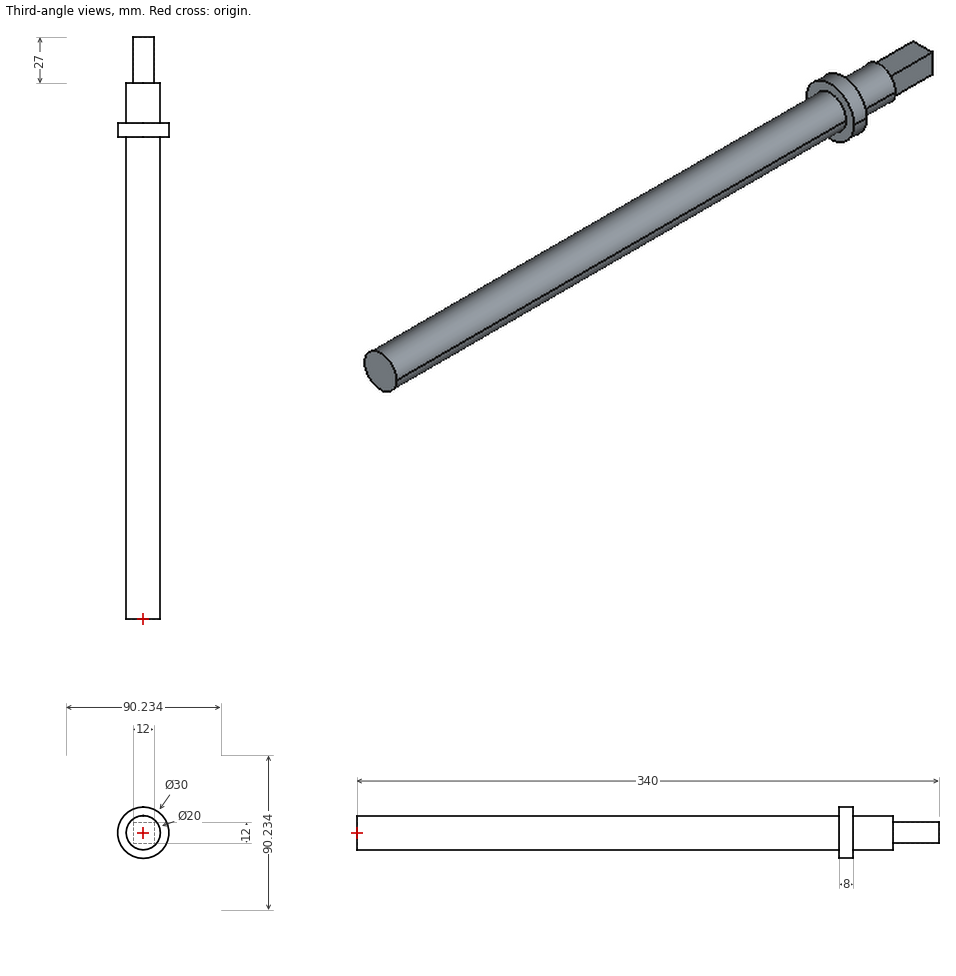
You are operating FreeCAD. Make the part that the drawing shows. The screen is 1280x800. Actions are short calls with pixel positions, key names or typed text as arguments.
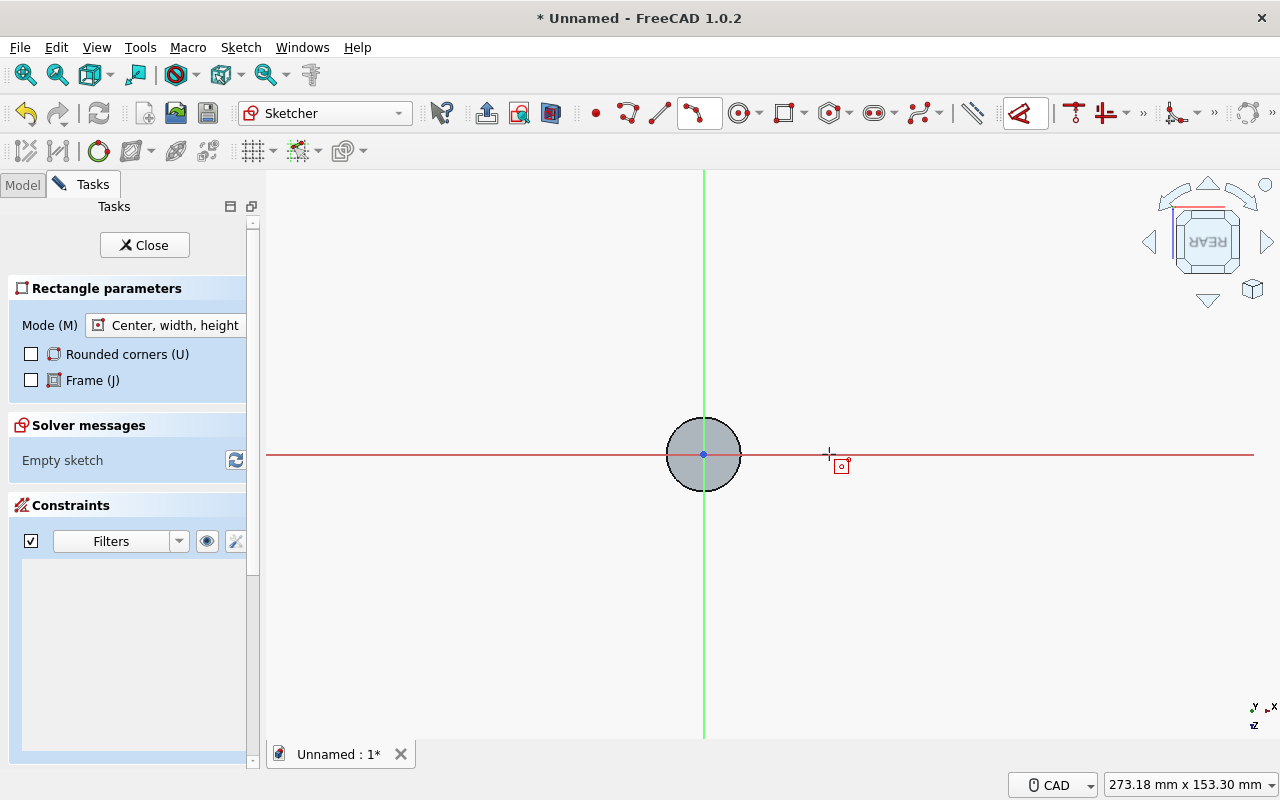
click(704, 454)
move(871, 287)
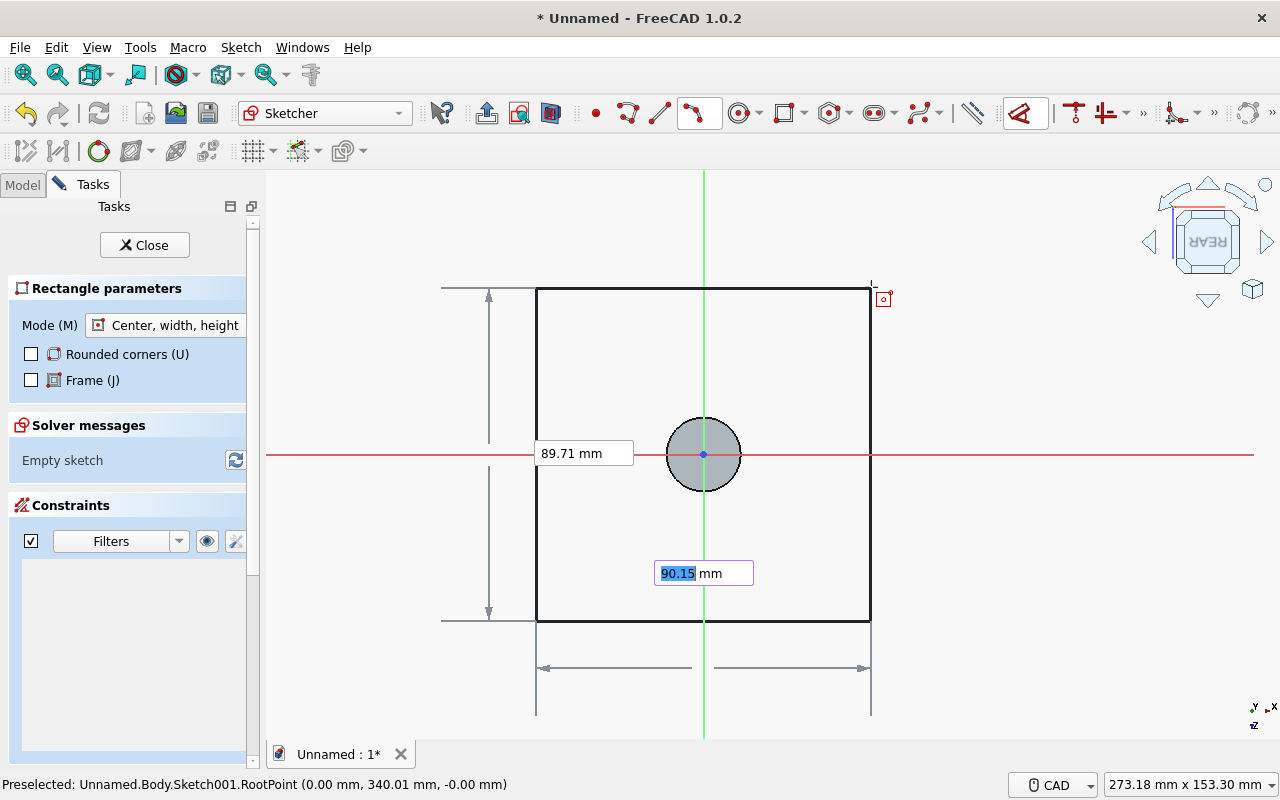
text(90.234)
key(Tab)
text(90.234)
key(Return)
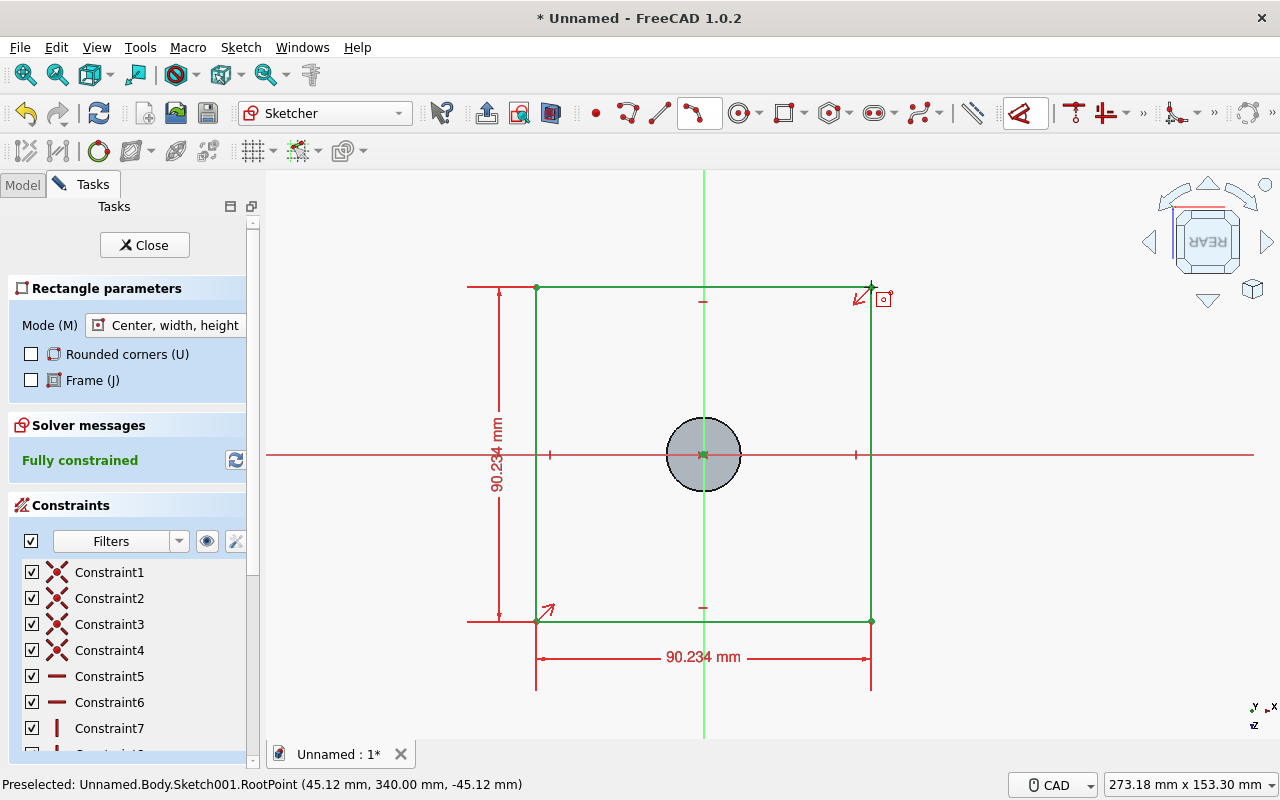
click(704, 454)
move(726, 432)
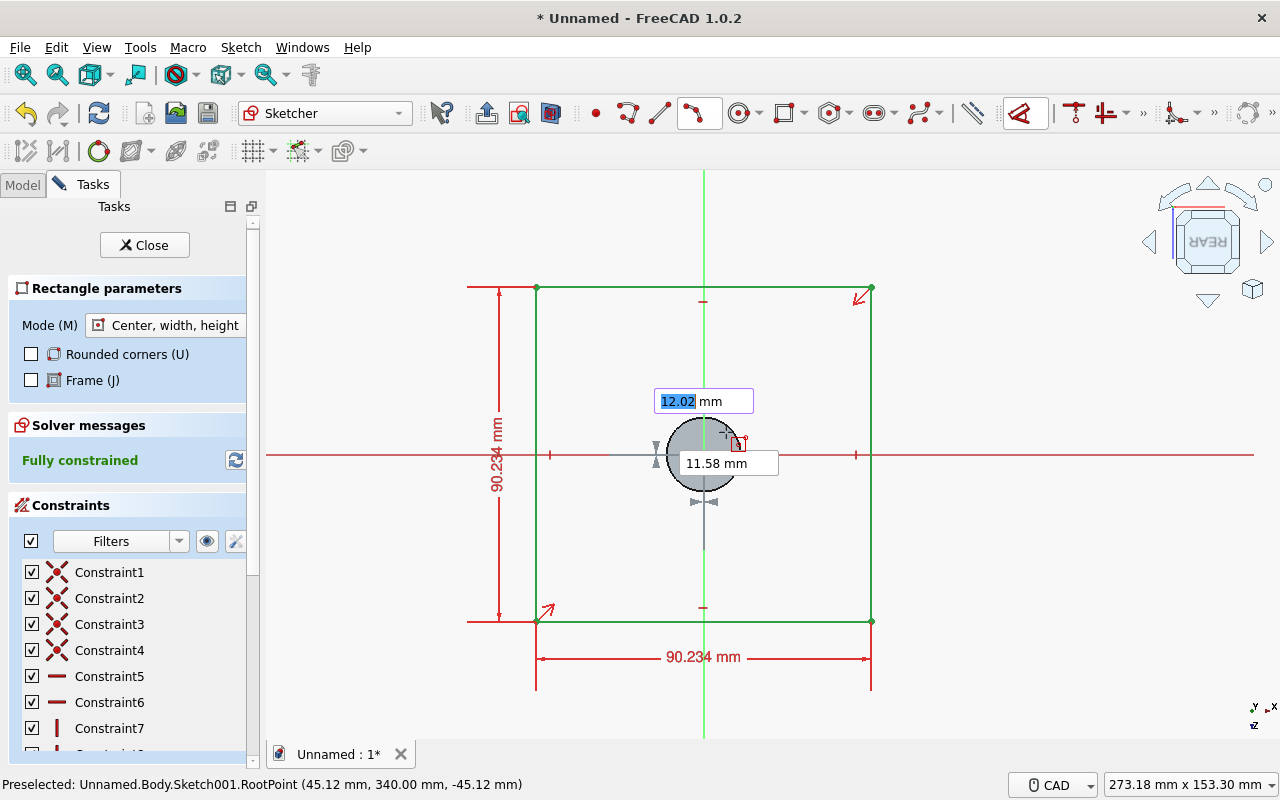
text(12)
key(Tab)
text(12)
key(Return)
key(Escape)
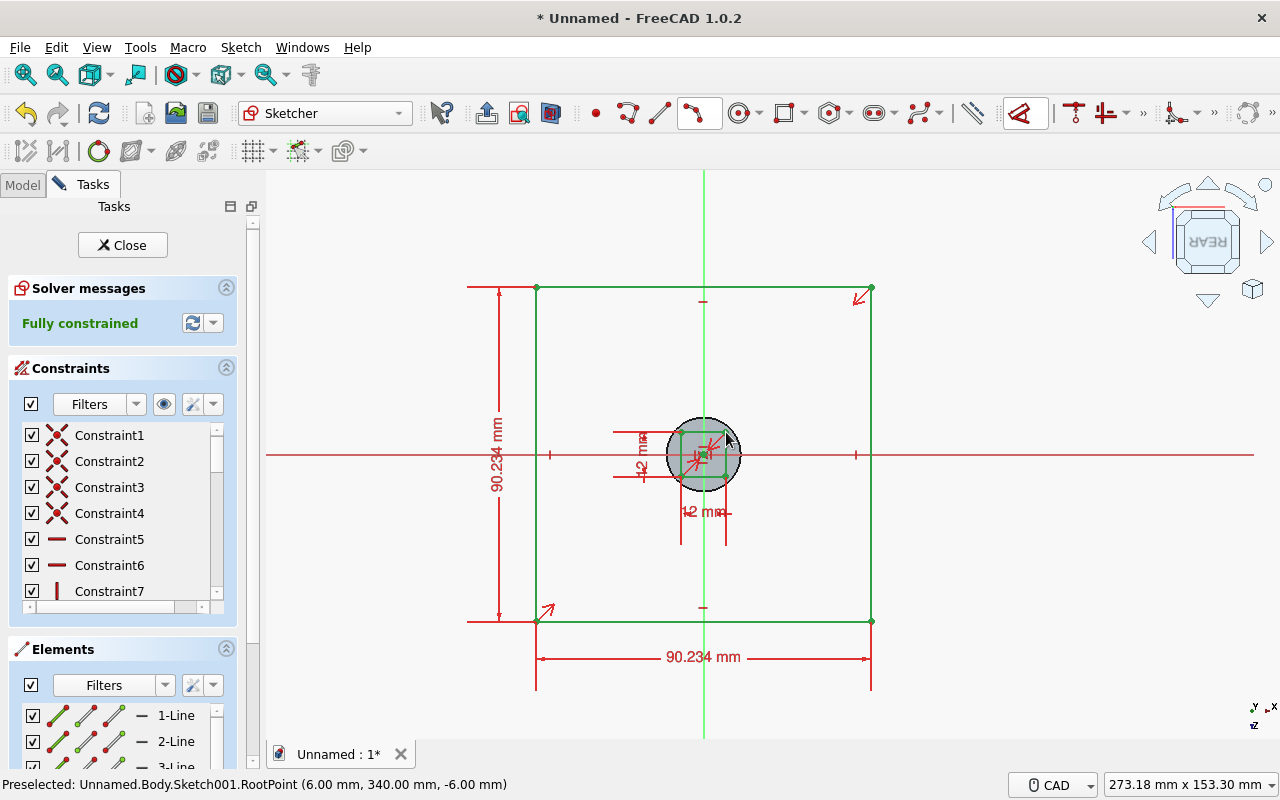
click(123, 245)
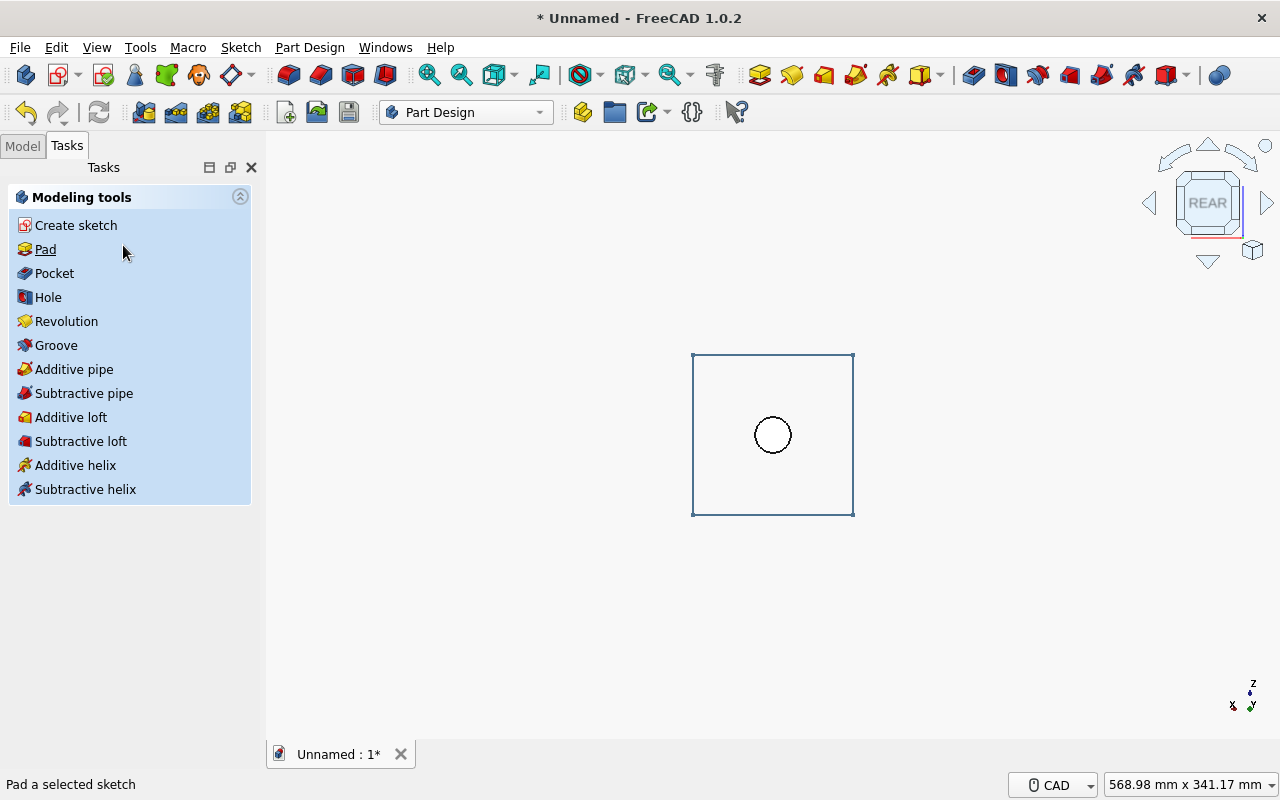
click(974, 76)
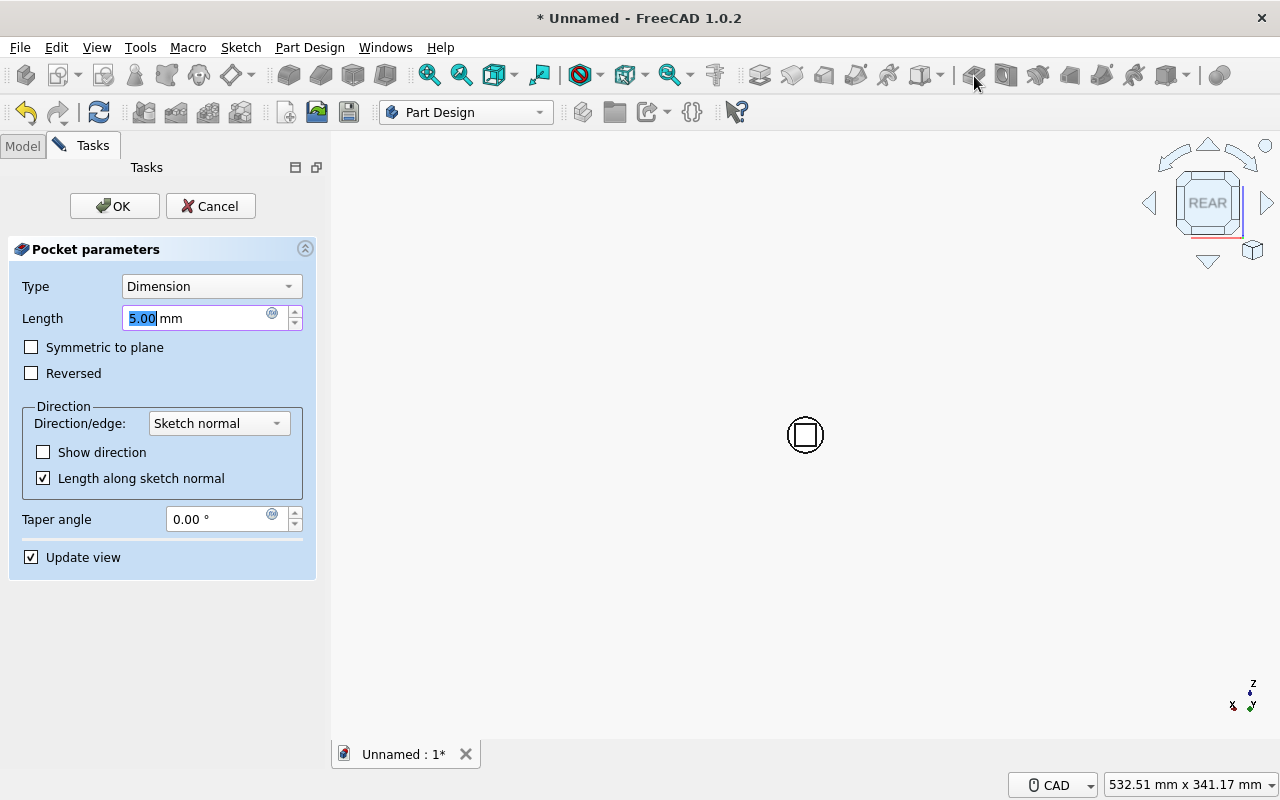
text(27)
key(Tab)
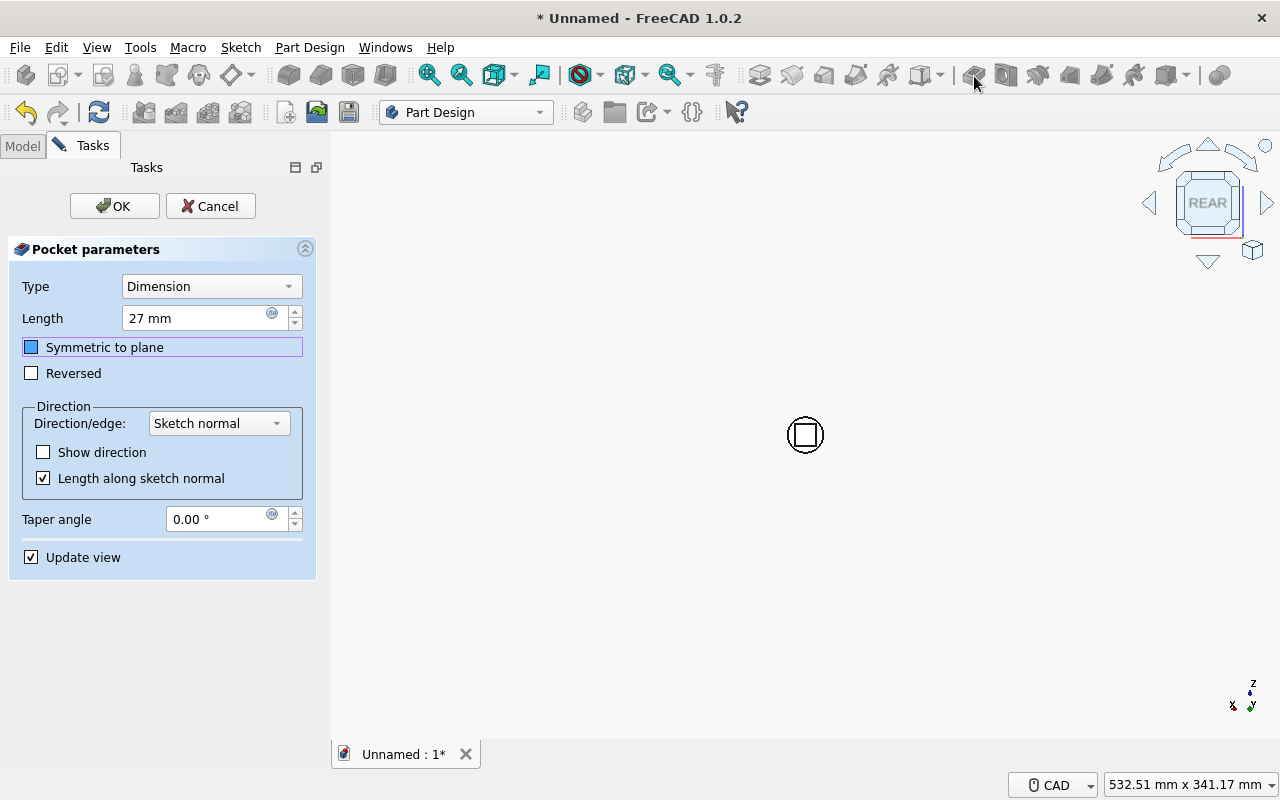
click(115, 206)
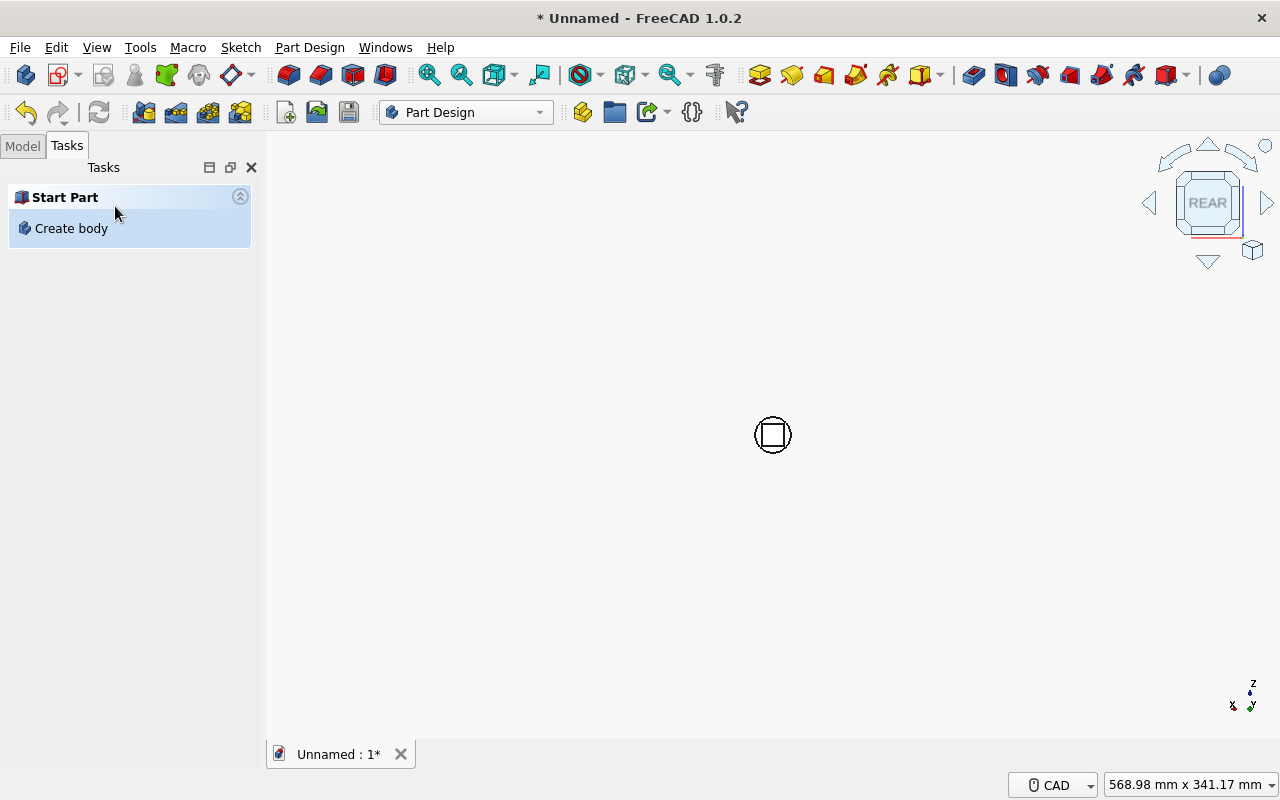
key(v)
key(f)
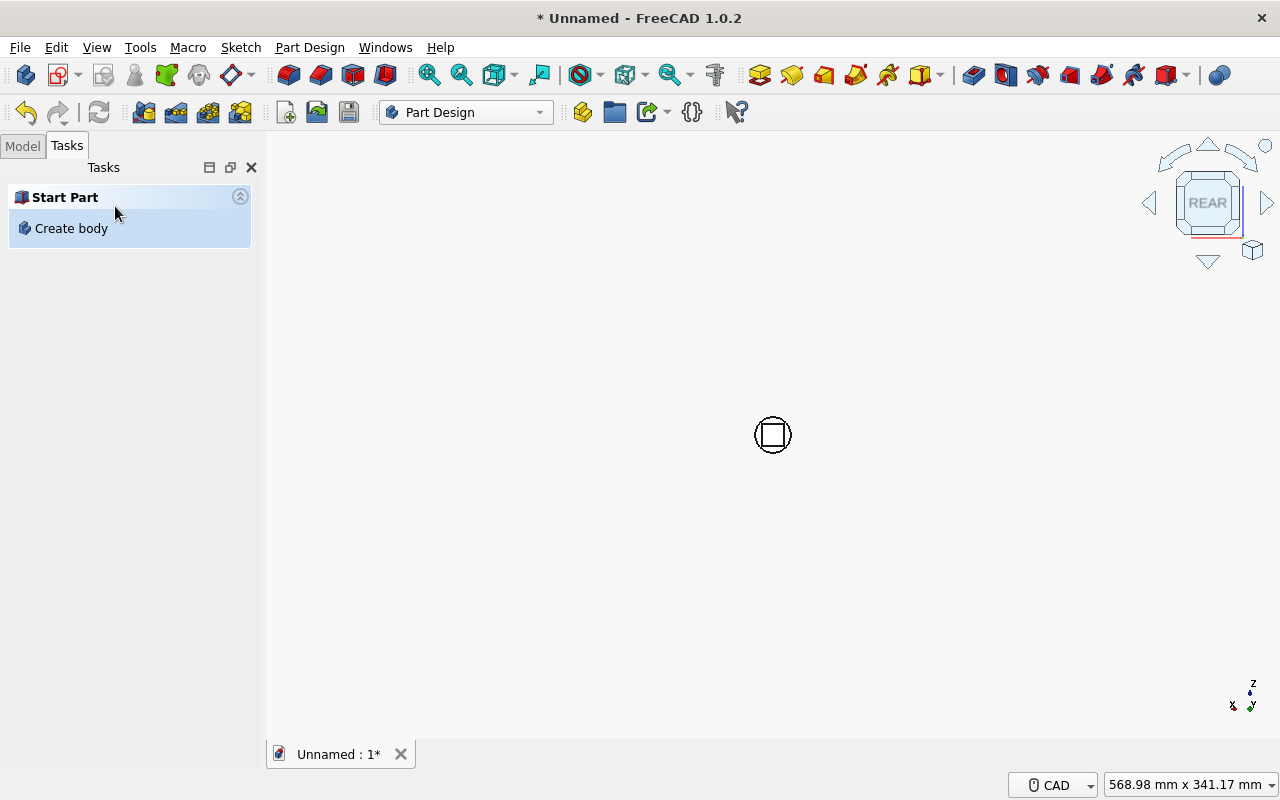
click(23, 145)